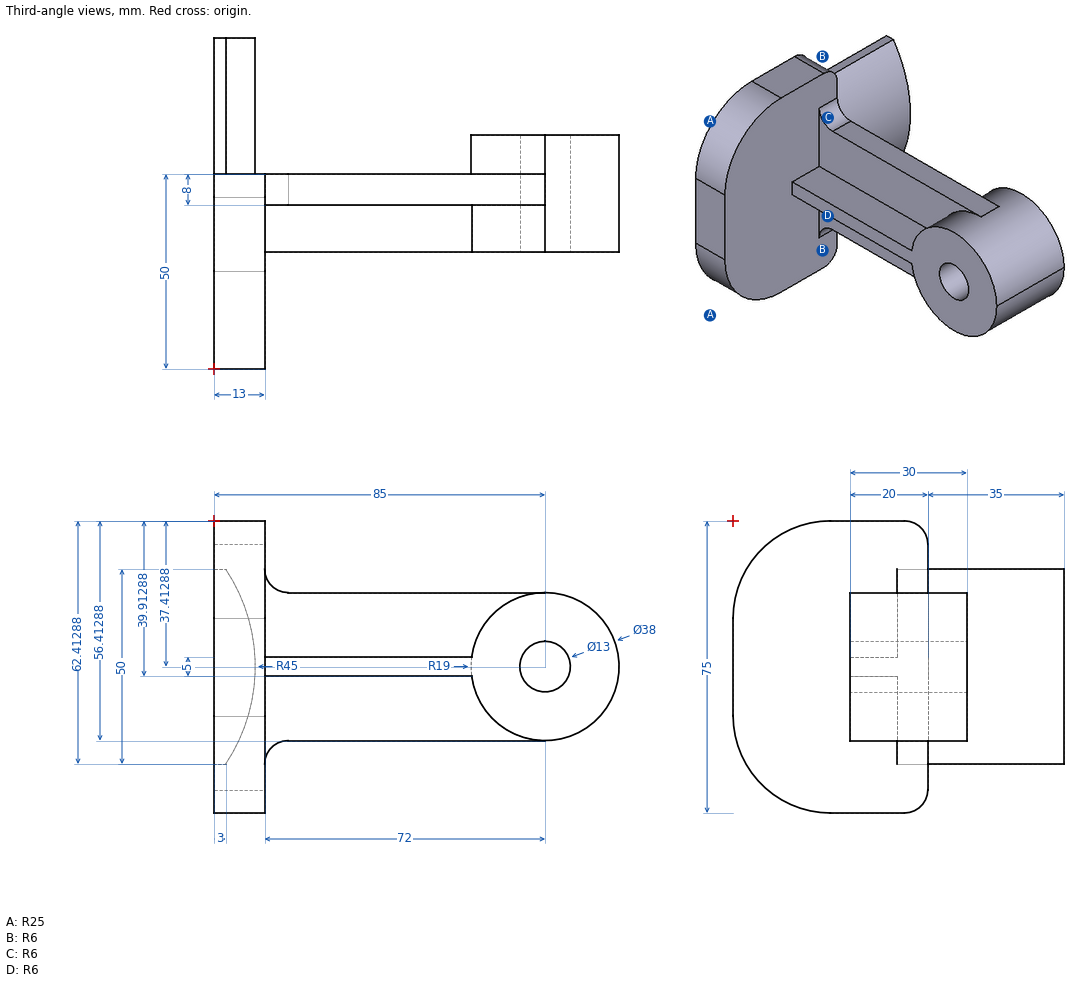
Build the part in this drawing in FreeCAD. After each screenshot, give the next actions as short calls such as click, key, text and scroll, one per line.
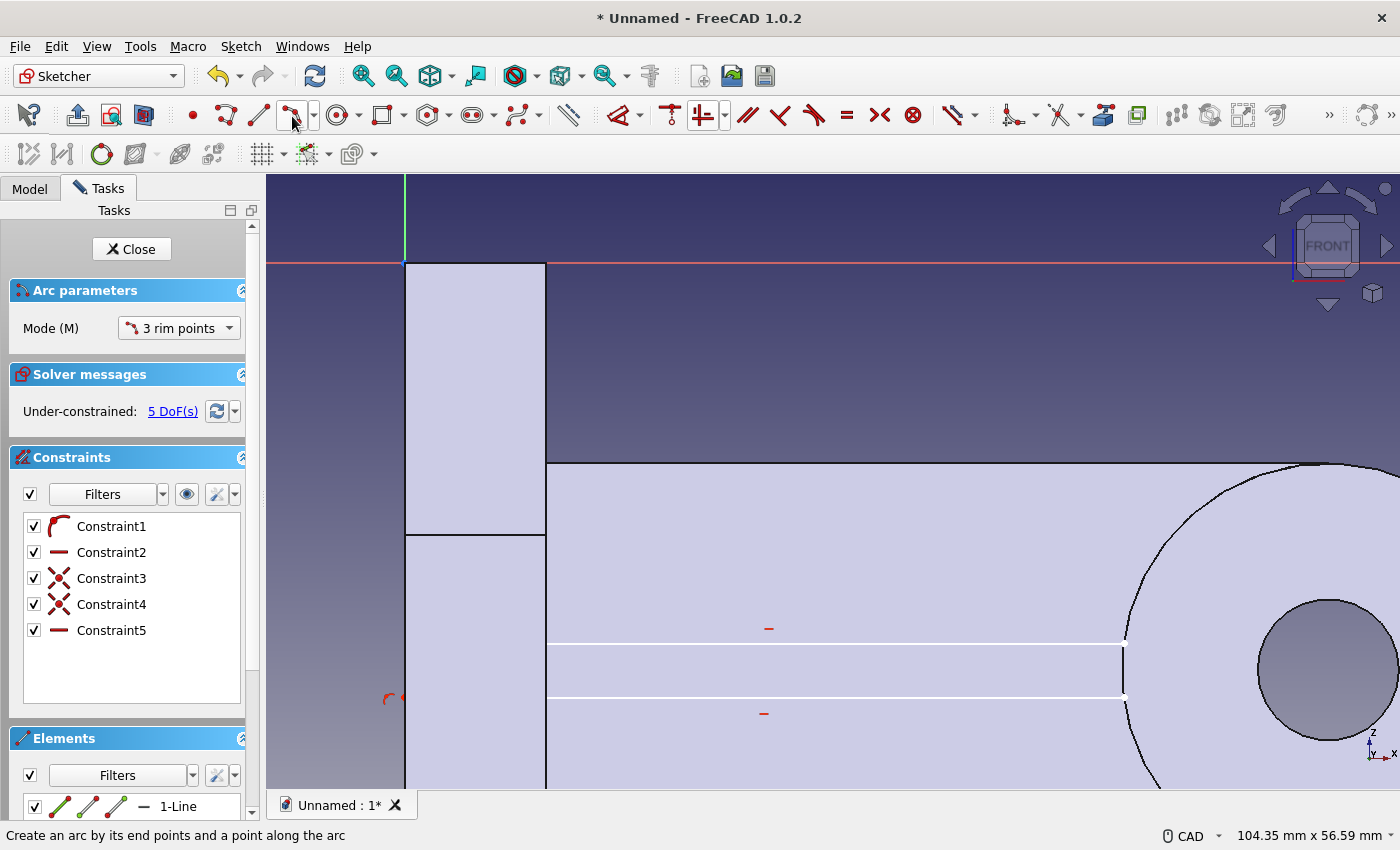
click(1124, 644)
click(1124, 698)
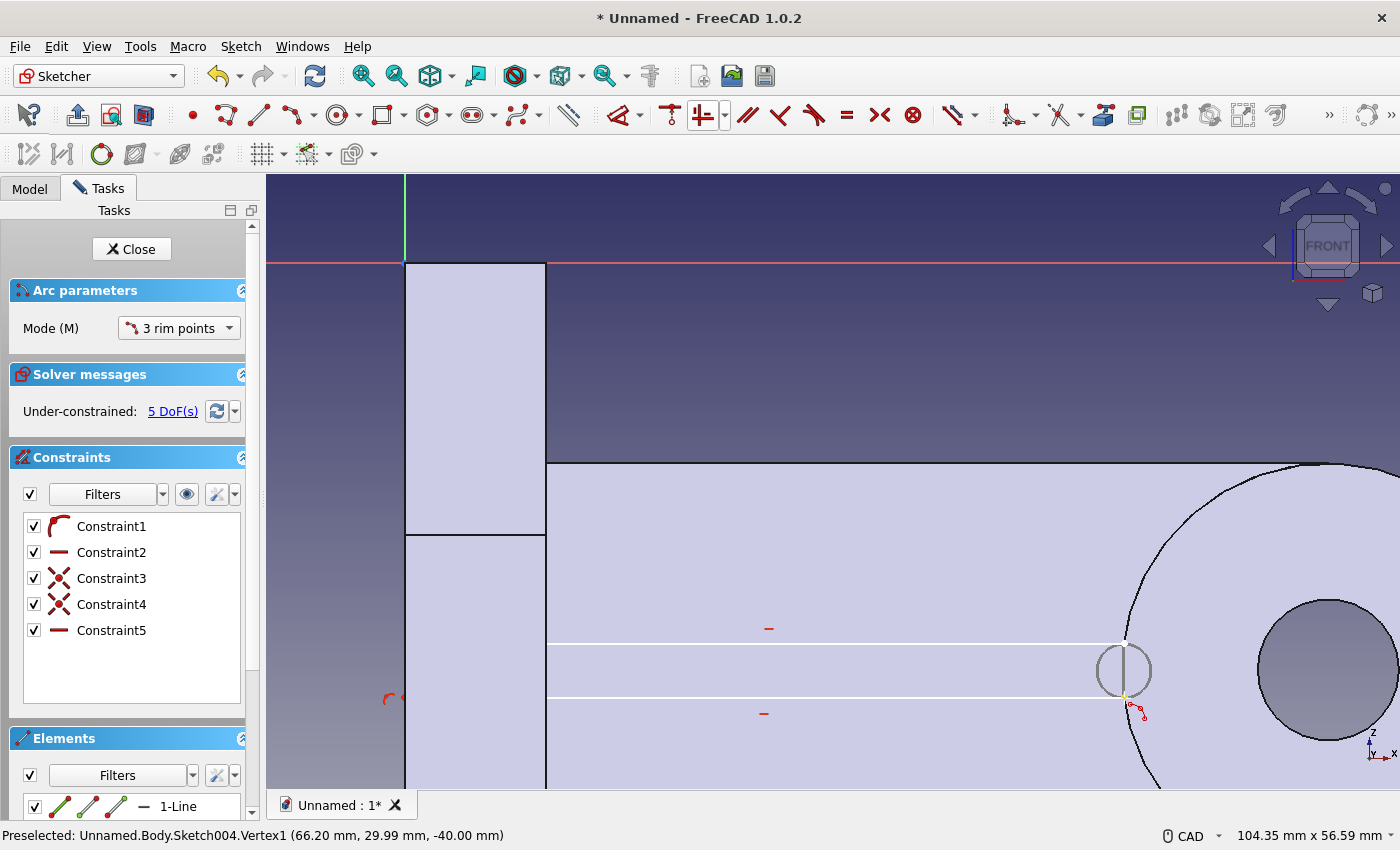
scroll(1122, 670, up, 11)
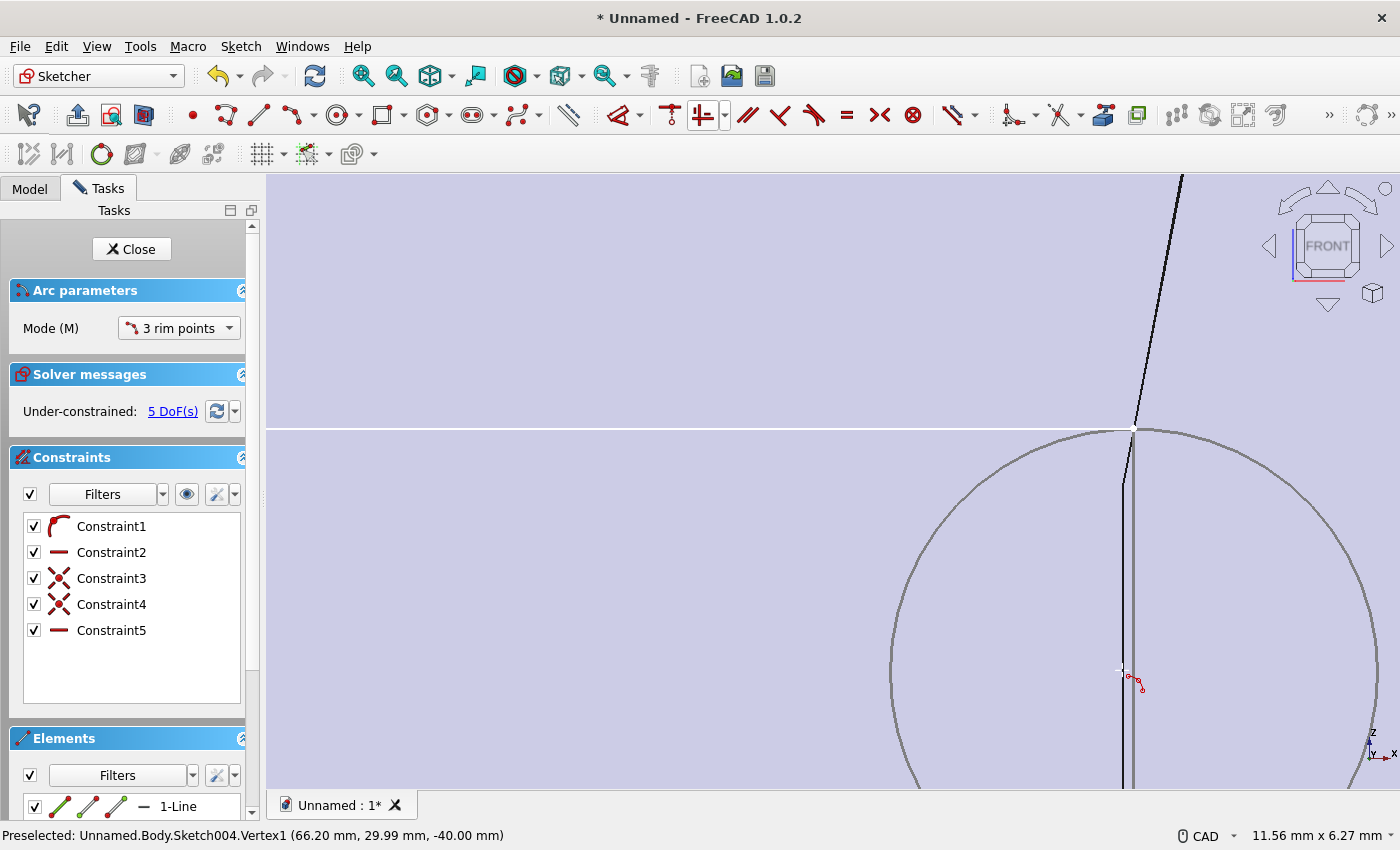
click(1115, 662)
key(Escape)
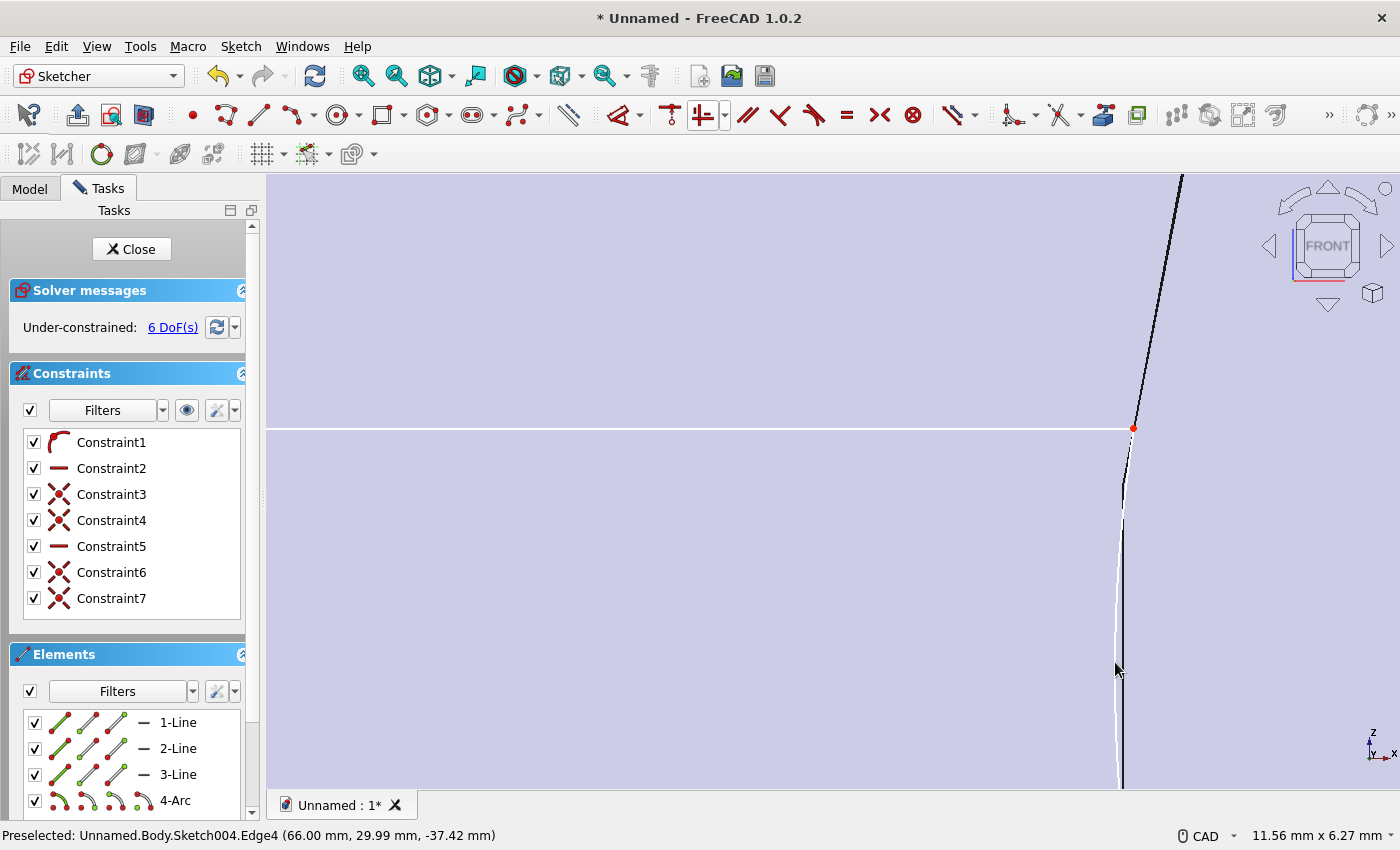
scroll(1123, 672, down, 11)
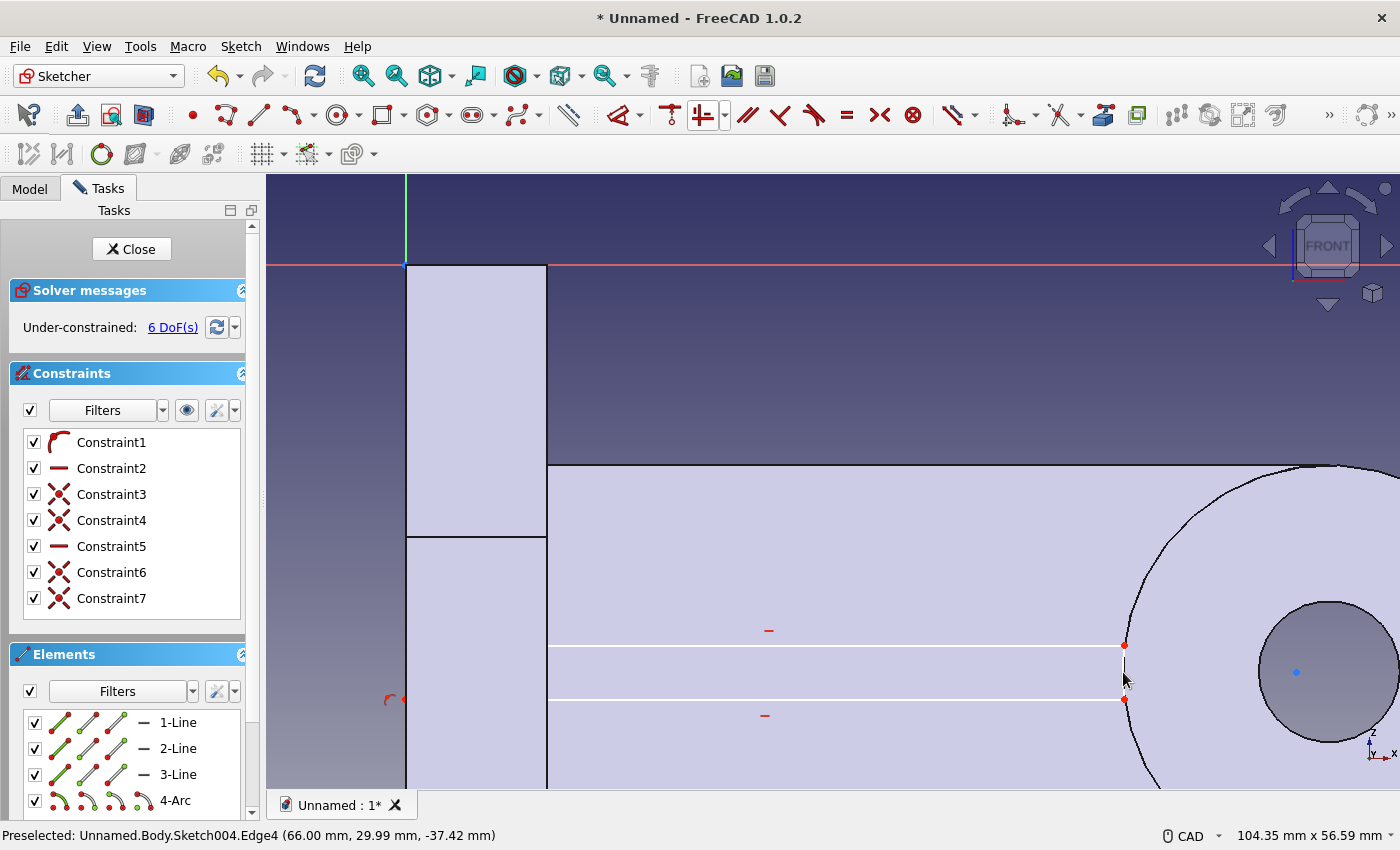
scroll(408, 684, up, 8)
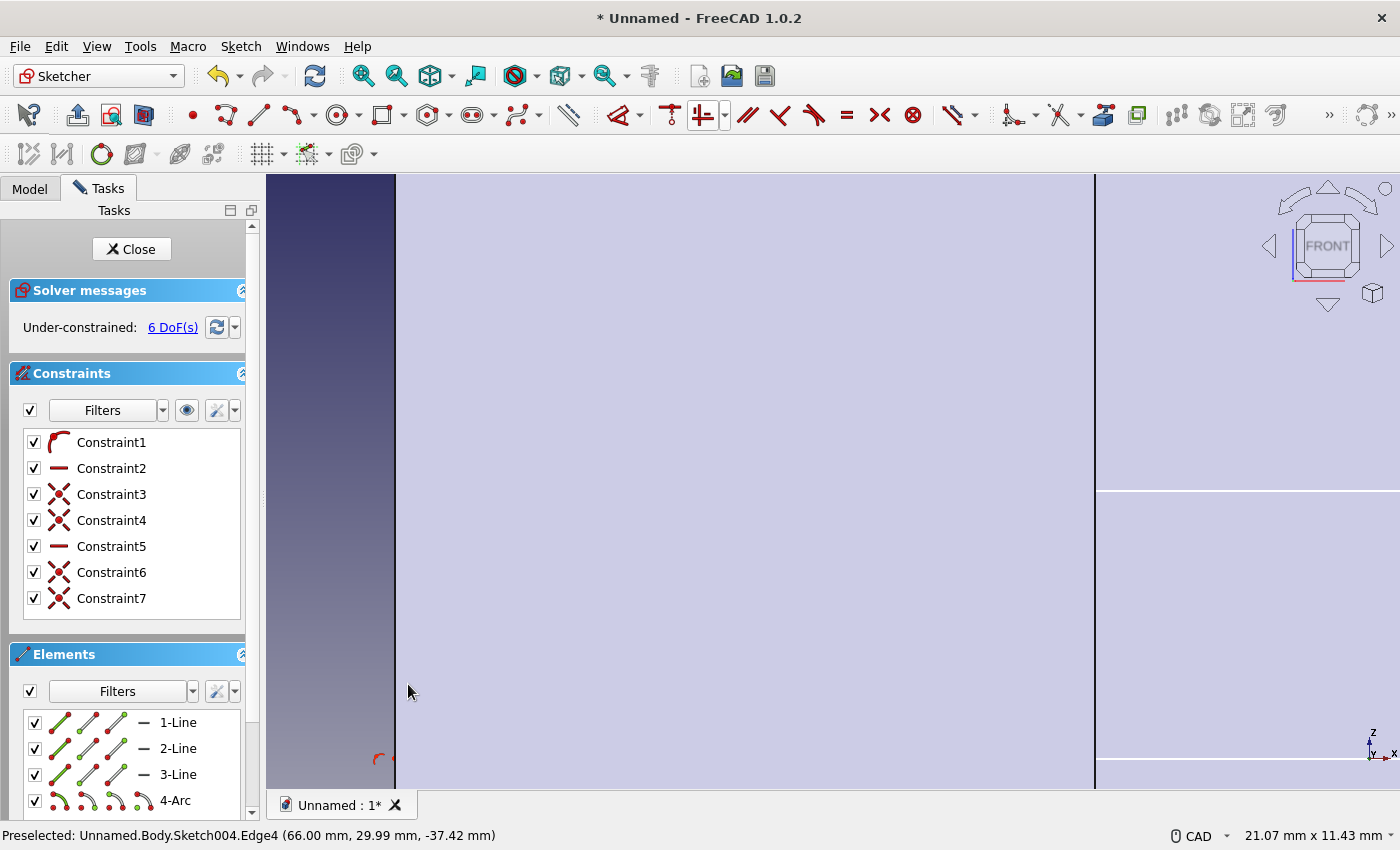
click(409, 679)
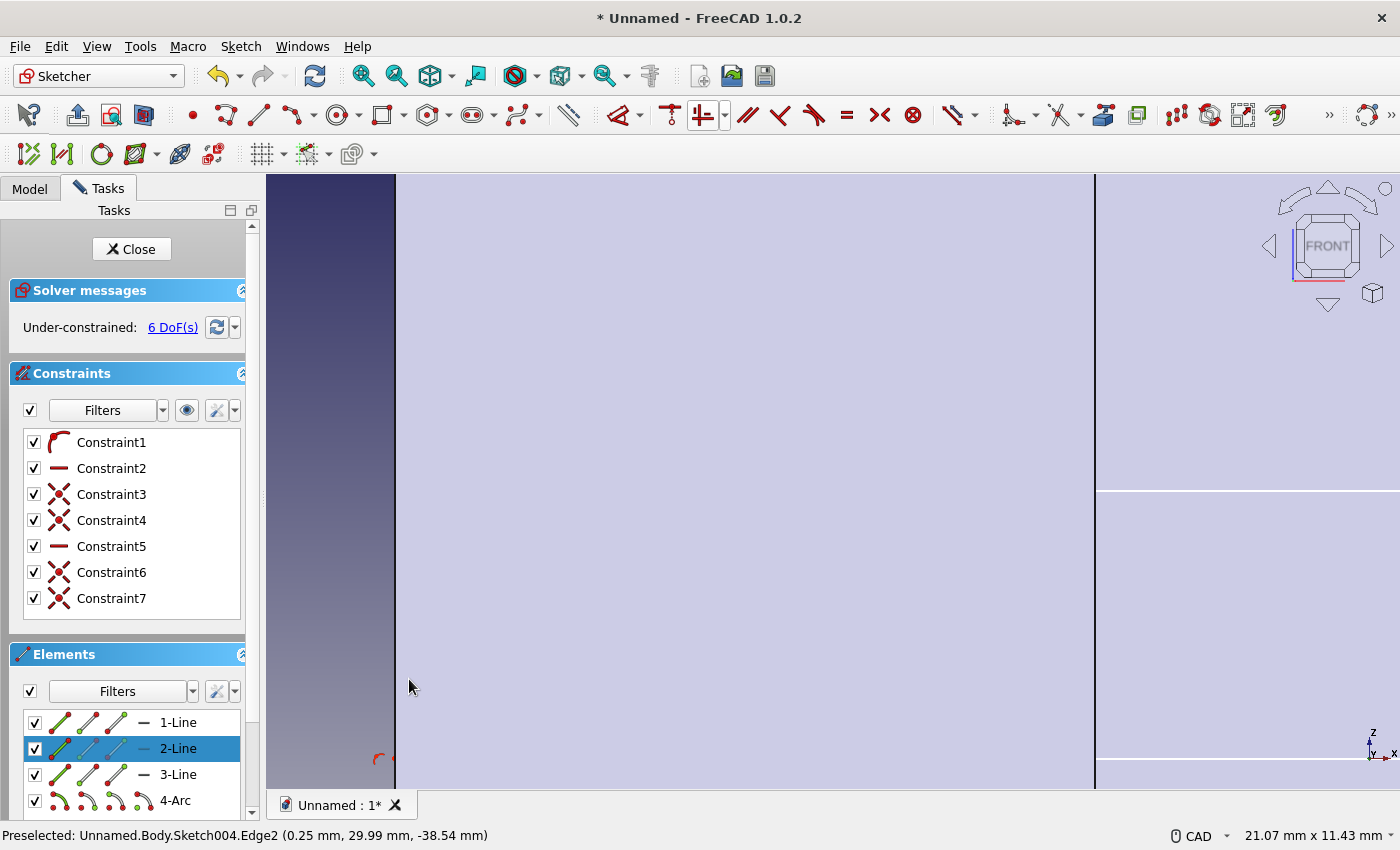
click(724, 116)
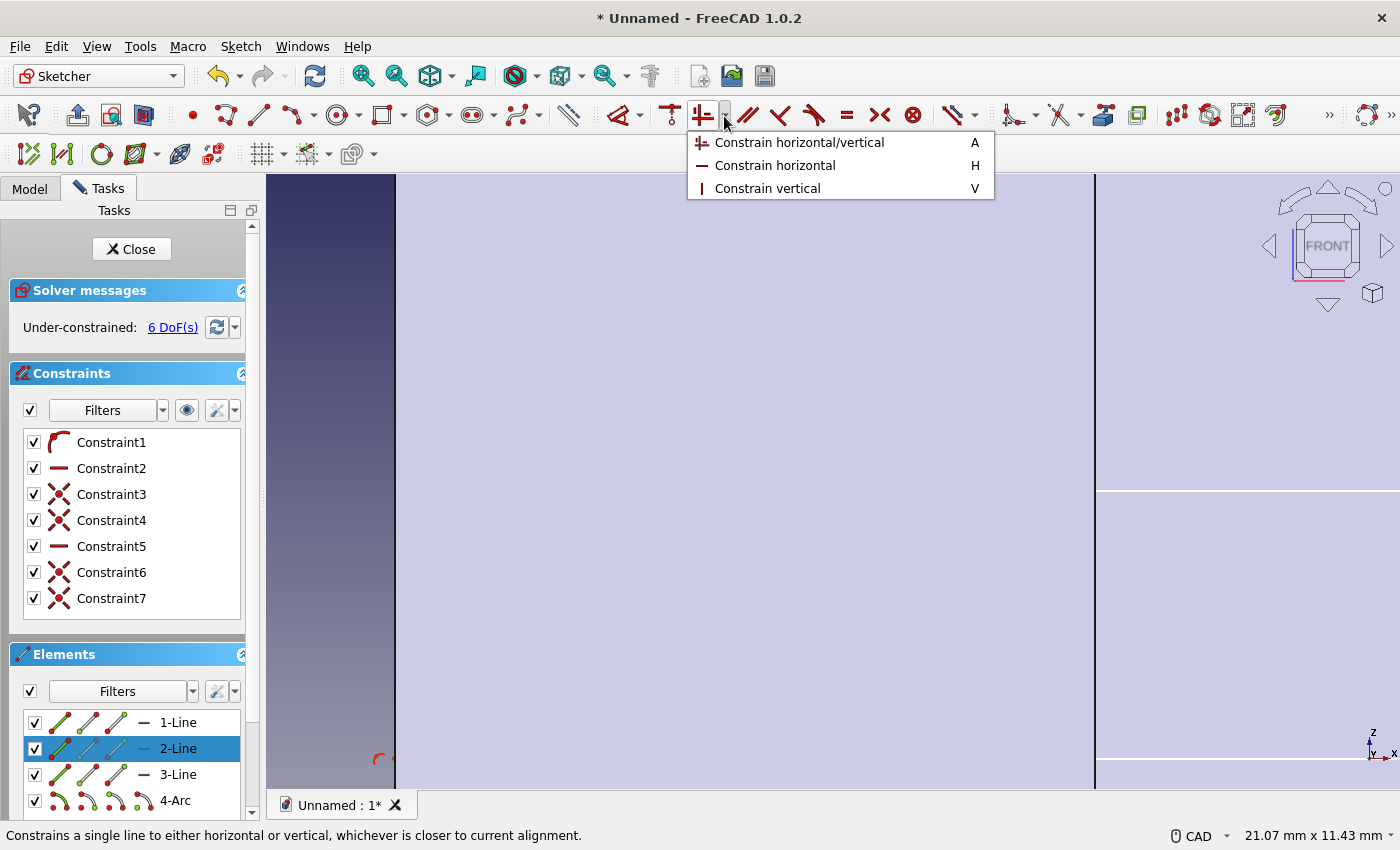
click(841, 188)